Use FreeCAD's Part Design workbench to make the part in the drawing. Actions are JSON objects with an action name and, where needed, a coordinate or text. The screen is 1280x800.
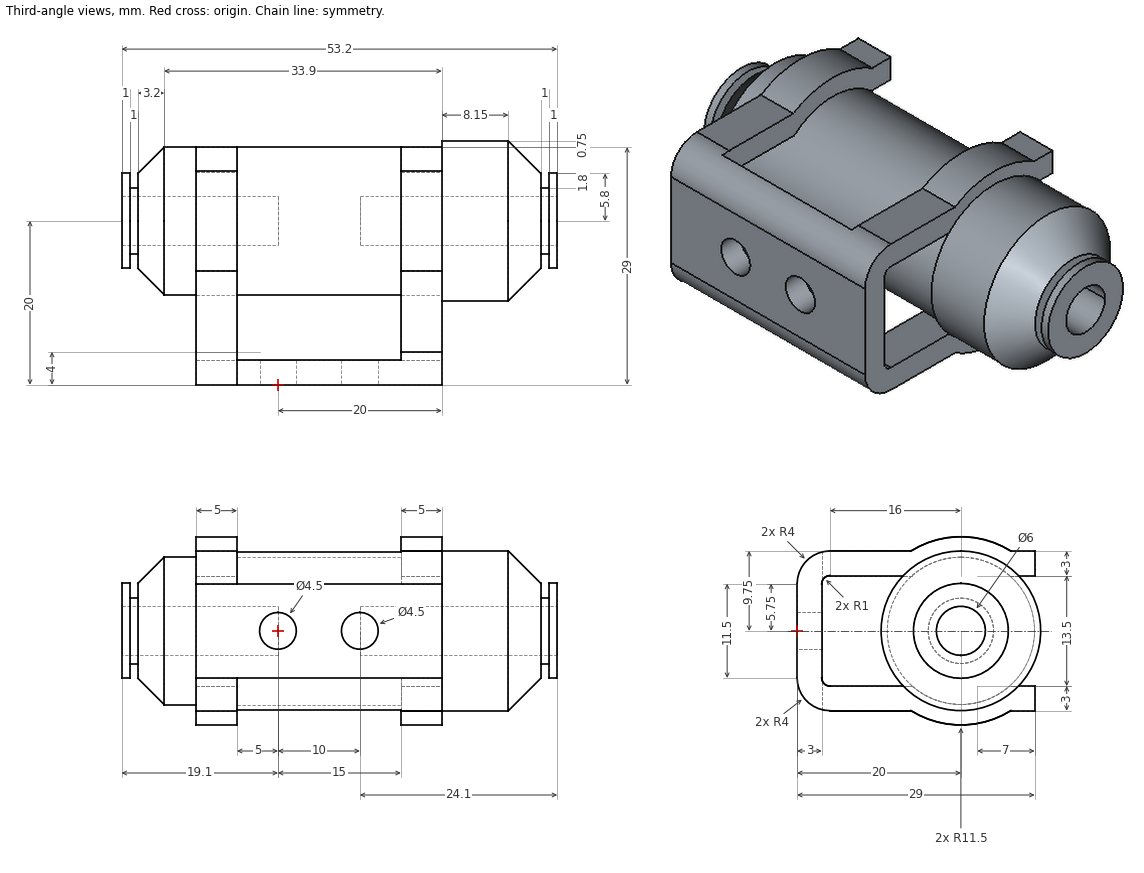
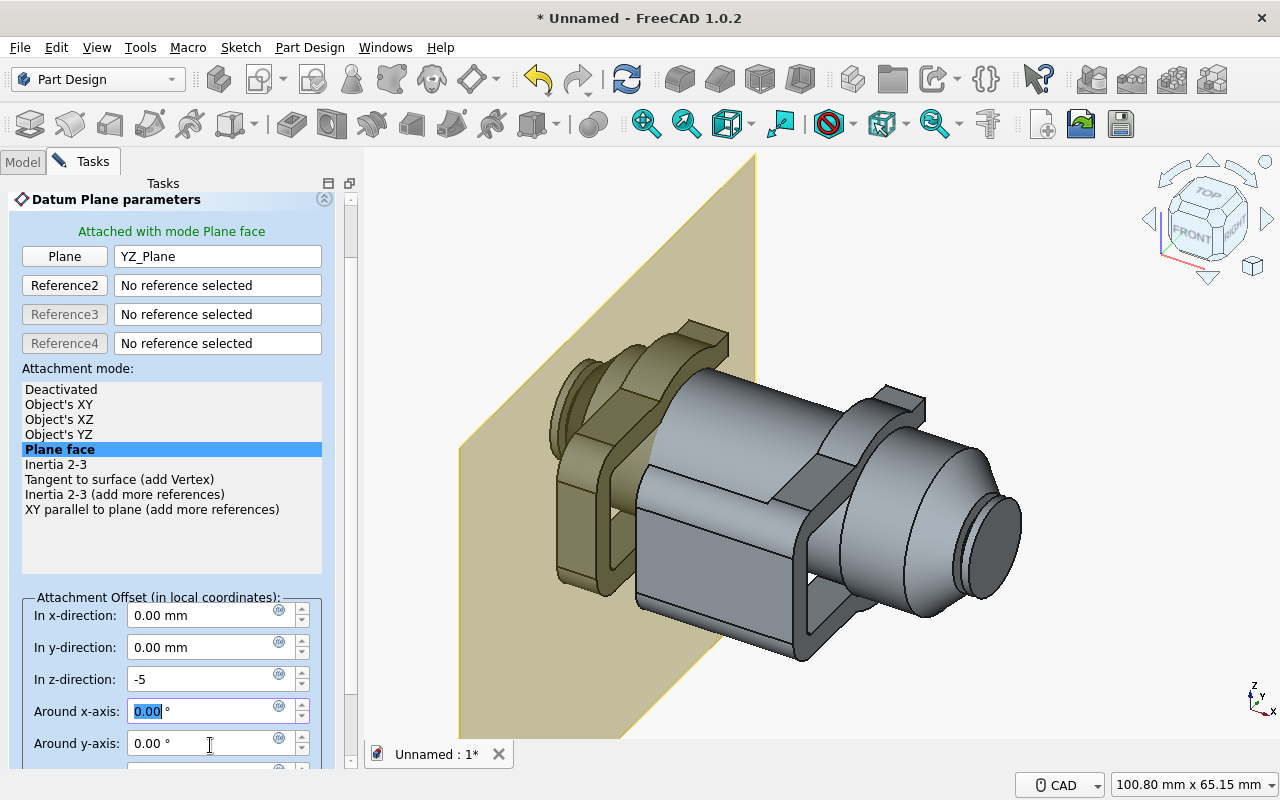
{"action": "scroll", "coordinate": [351, 480], "scroll_direction": "up", "scroll_amount": 2}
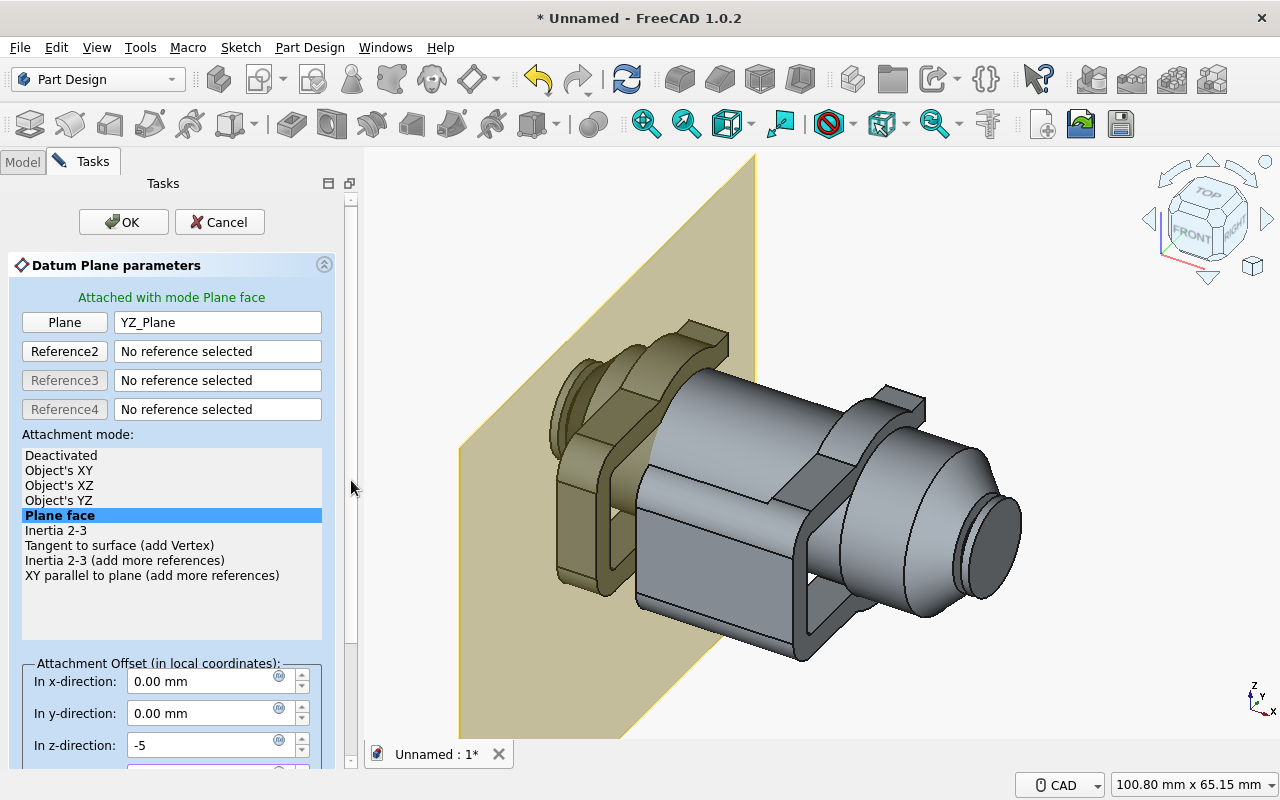
{"action": "left_click", "coordinate": [124, 222]}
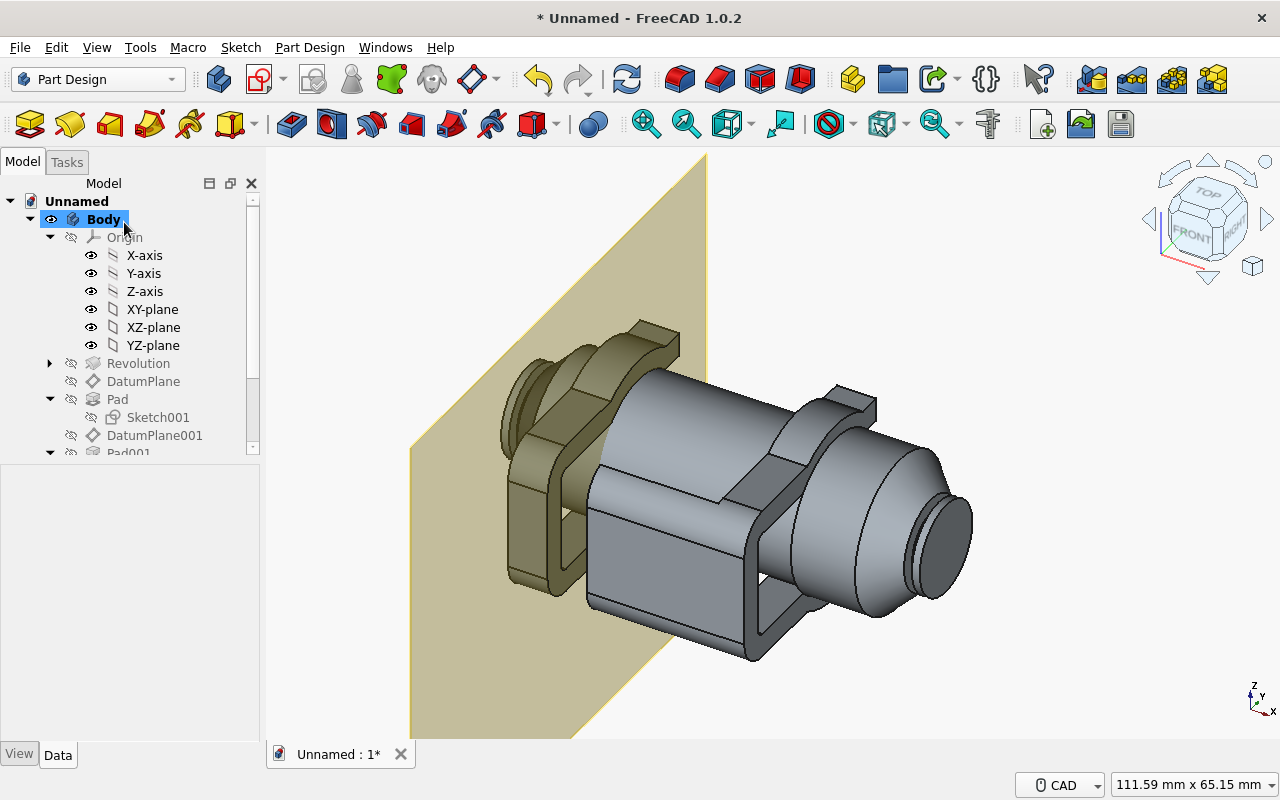
{"action": "scroll", "coordinate": [100, 323], "scroll_direction": "down", "scroll_amount": 3}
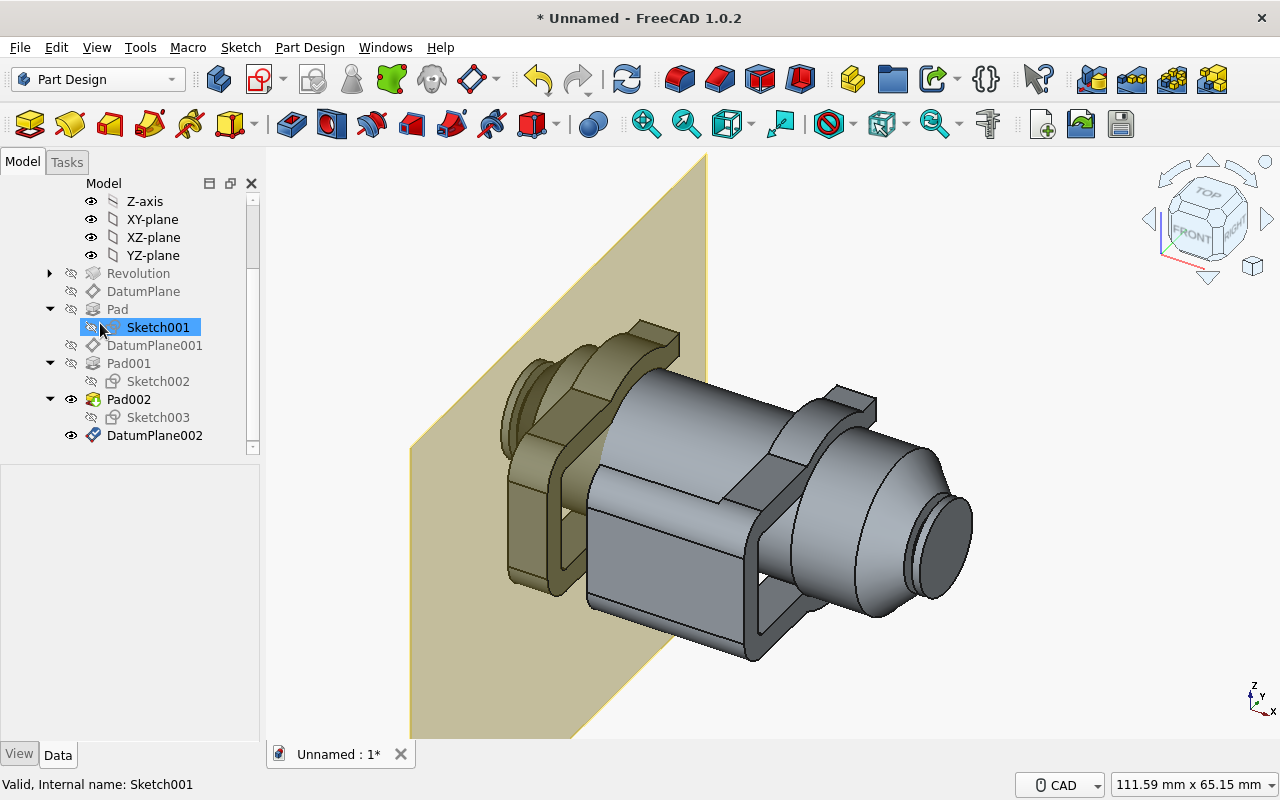
{"action": "left_click", "coordinate": [116, 435]}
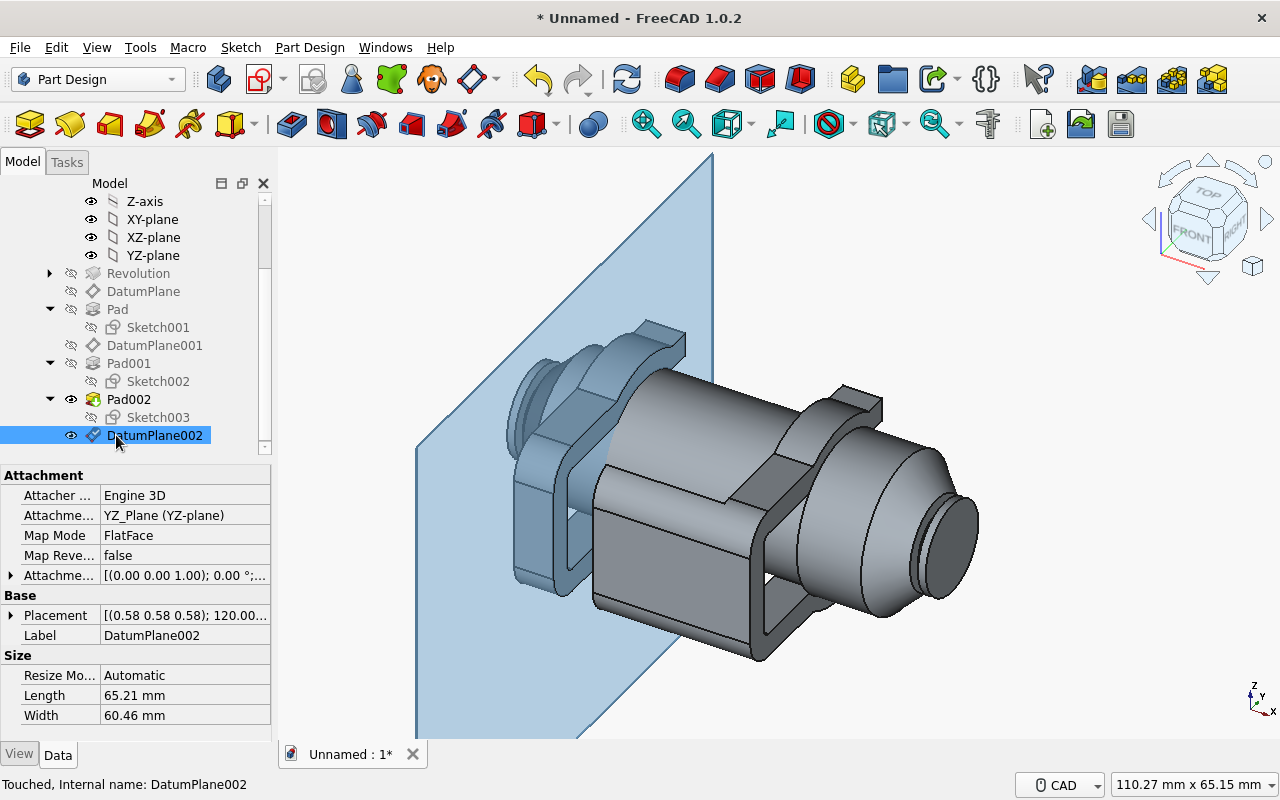
{"action": "left_click", "coordinate": [260, 80]}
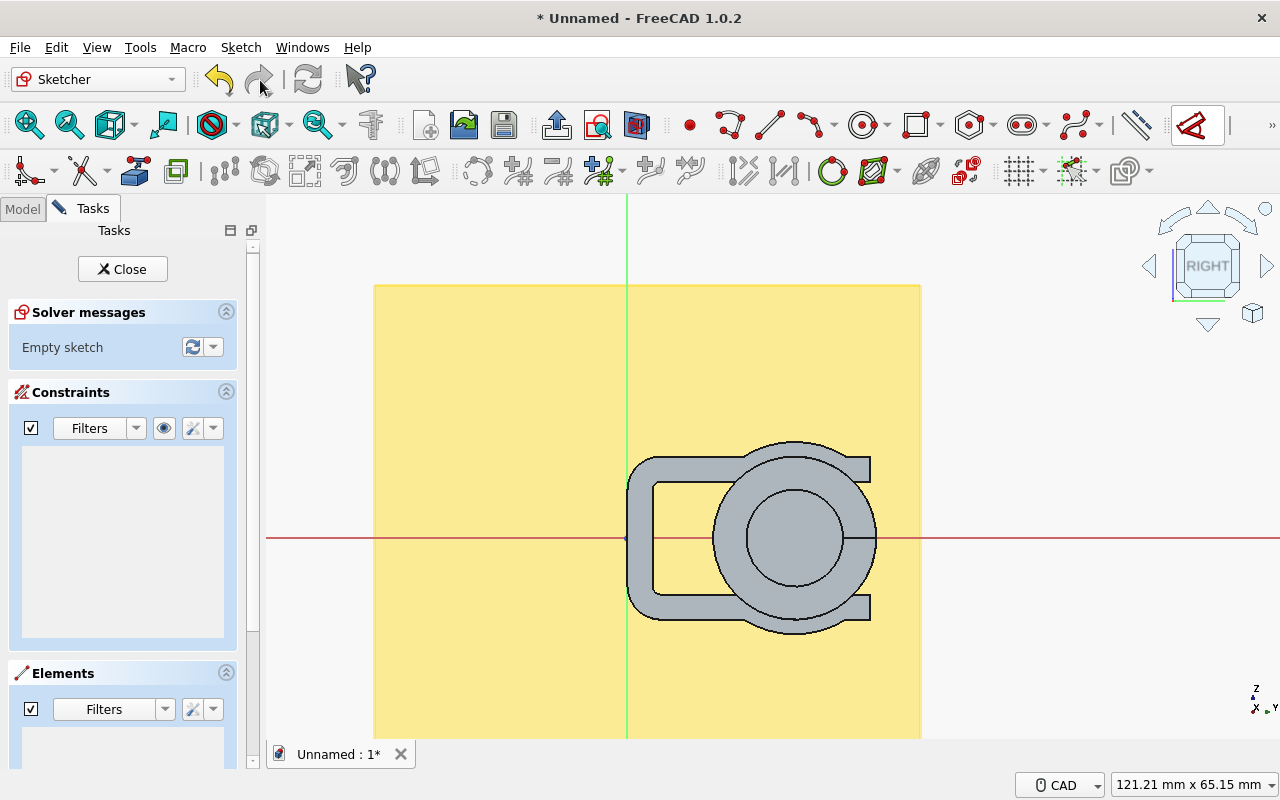
{"action": "left_click", "coordinate": [638, 126]}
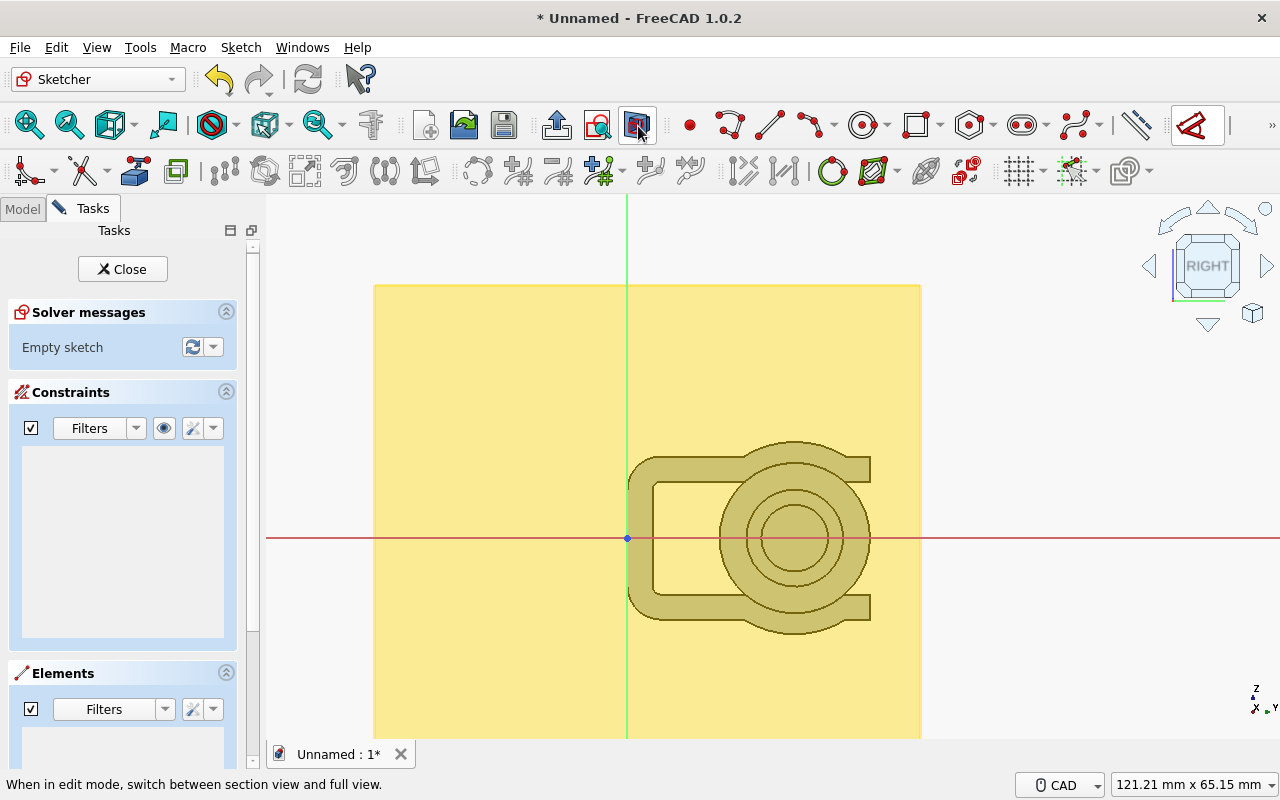
{"action": "scroll", "coordinate": [587, 597], "scroll_direction": "up", "scroll_amount": 4}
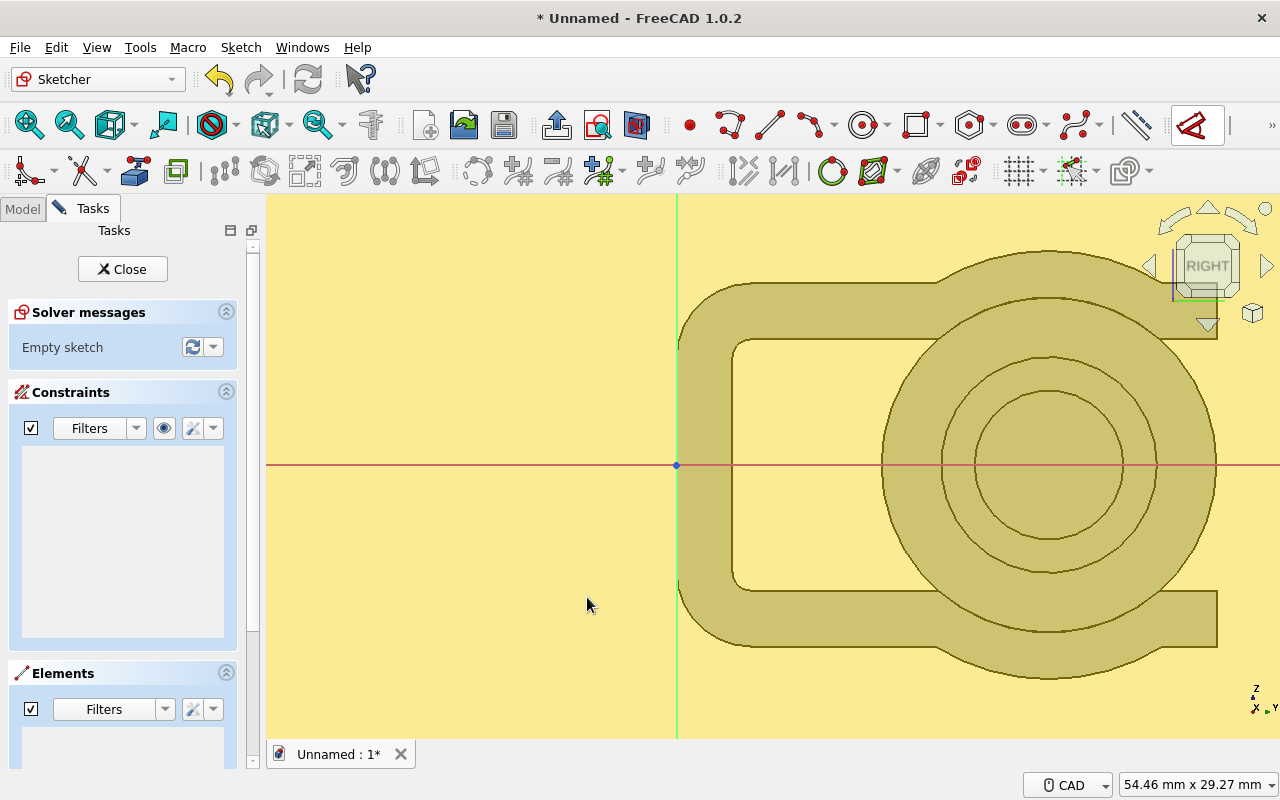
{"action": "left_click", "coordinate": [770, 126]}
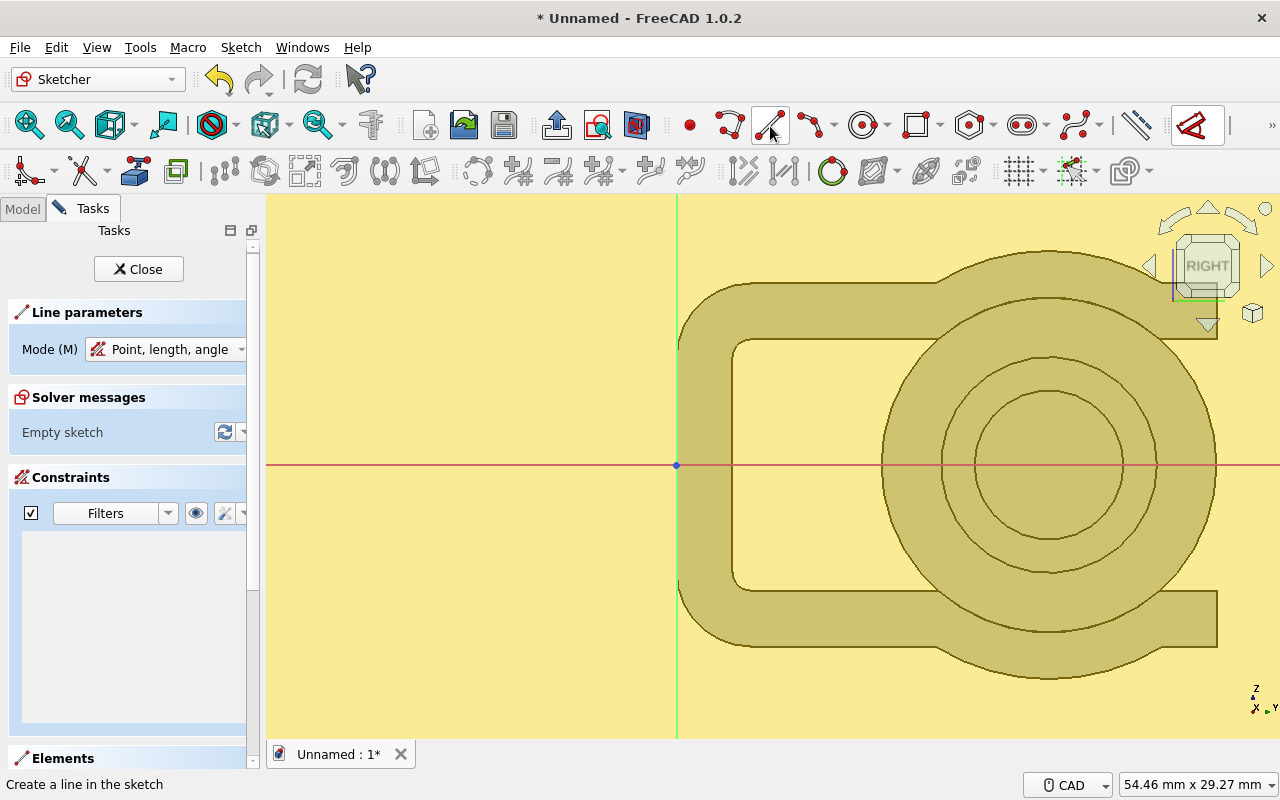
{"action": "left_click", "coordinate": [677, 358]}
{"action": "left_click", "coordinate": [686, 572]}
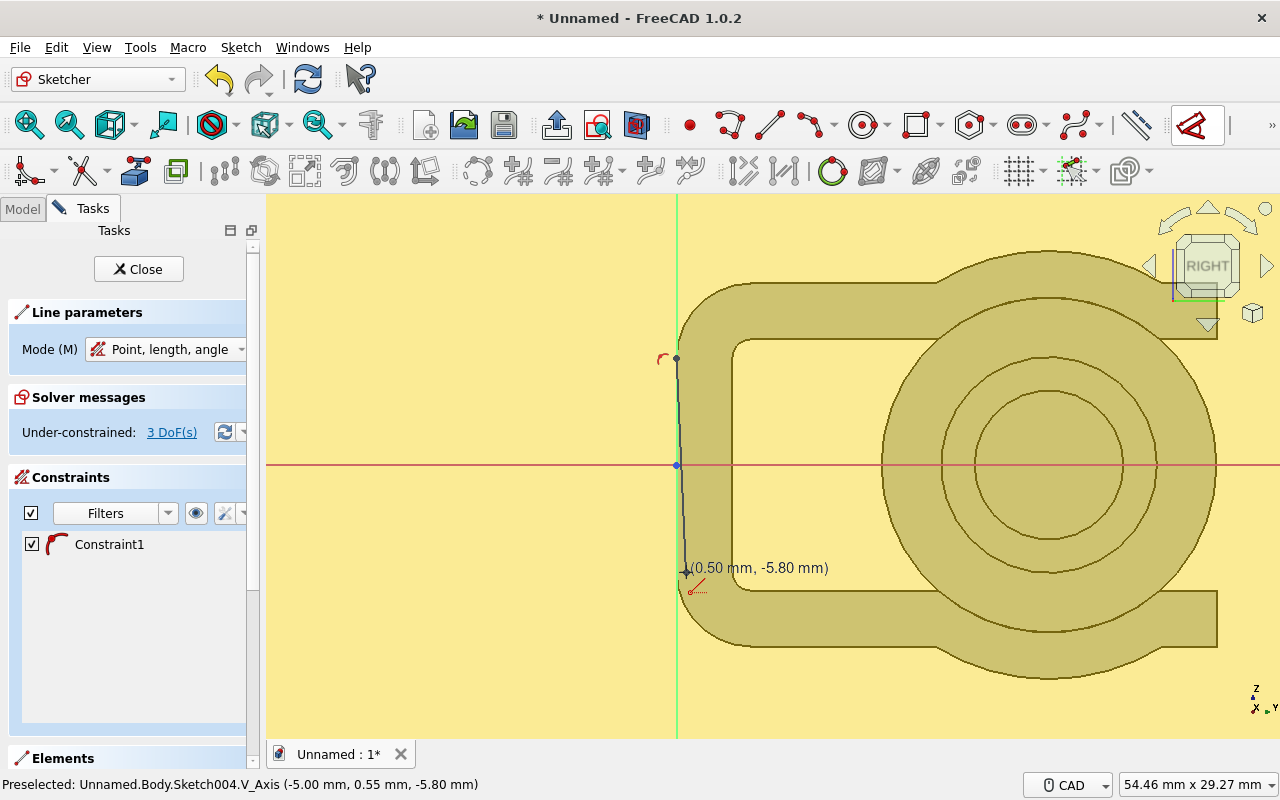
{"action": "left_click", "coordinate": [732, 644]}
{"action": "left_click", "coordinate": [732, 286]}